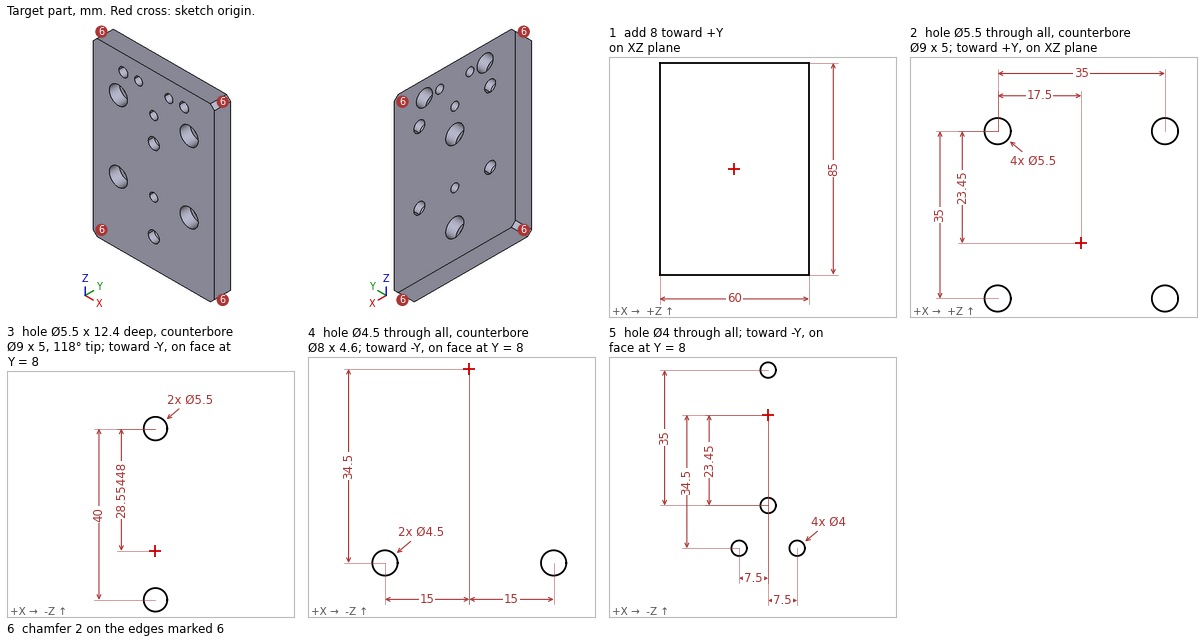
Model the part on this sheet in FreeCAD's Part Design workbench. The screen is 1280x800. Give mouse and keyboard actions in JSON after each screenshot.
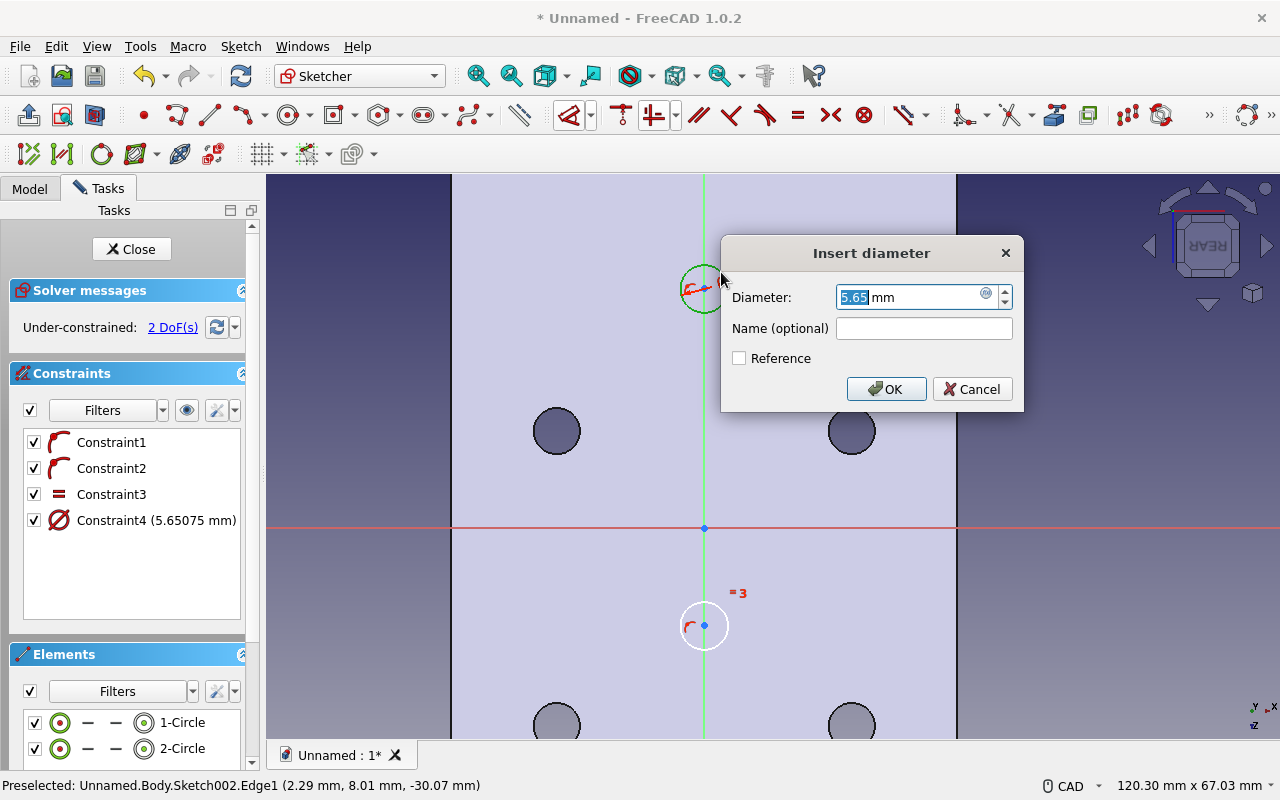
{"action": "type", "text": "5.5"}
{"action": "key", "text": "Return"}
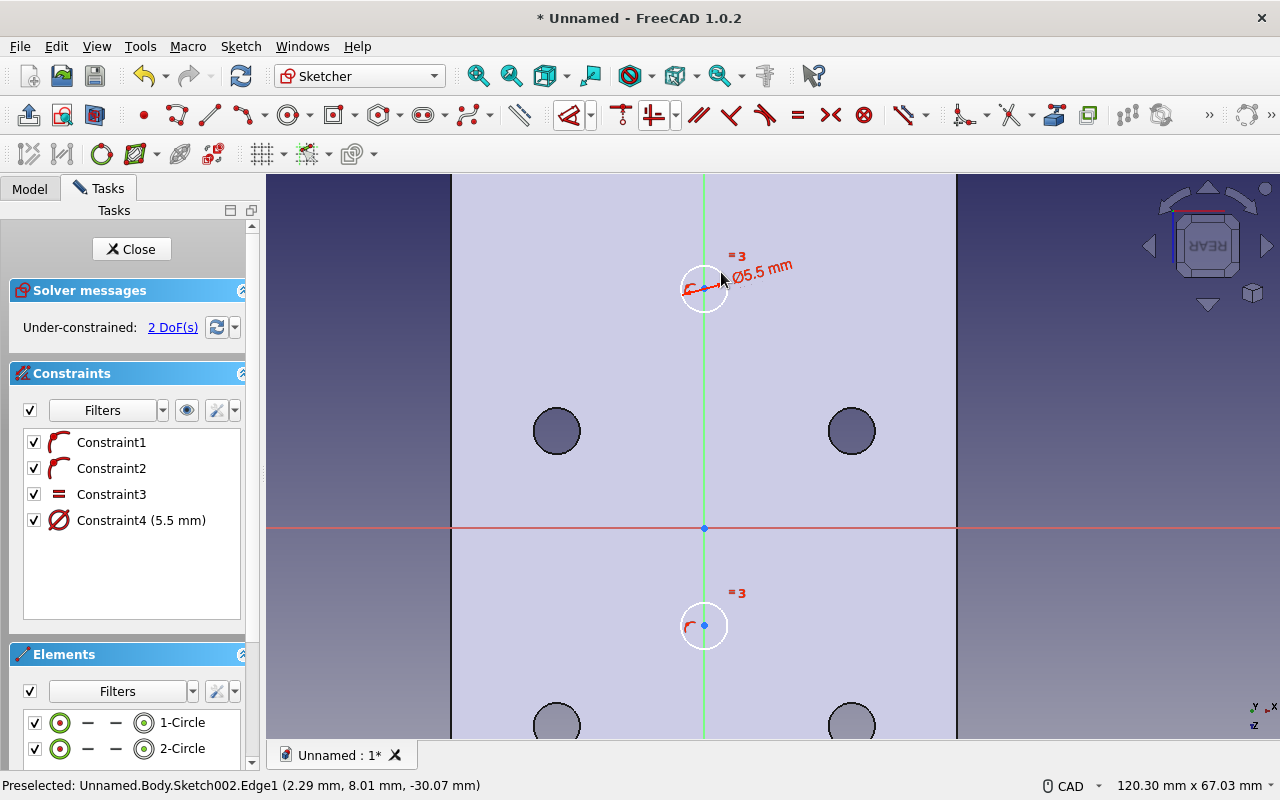
{"action": "left_click", "coordinate": [704, 289]}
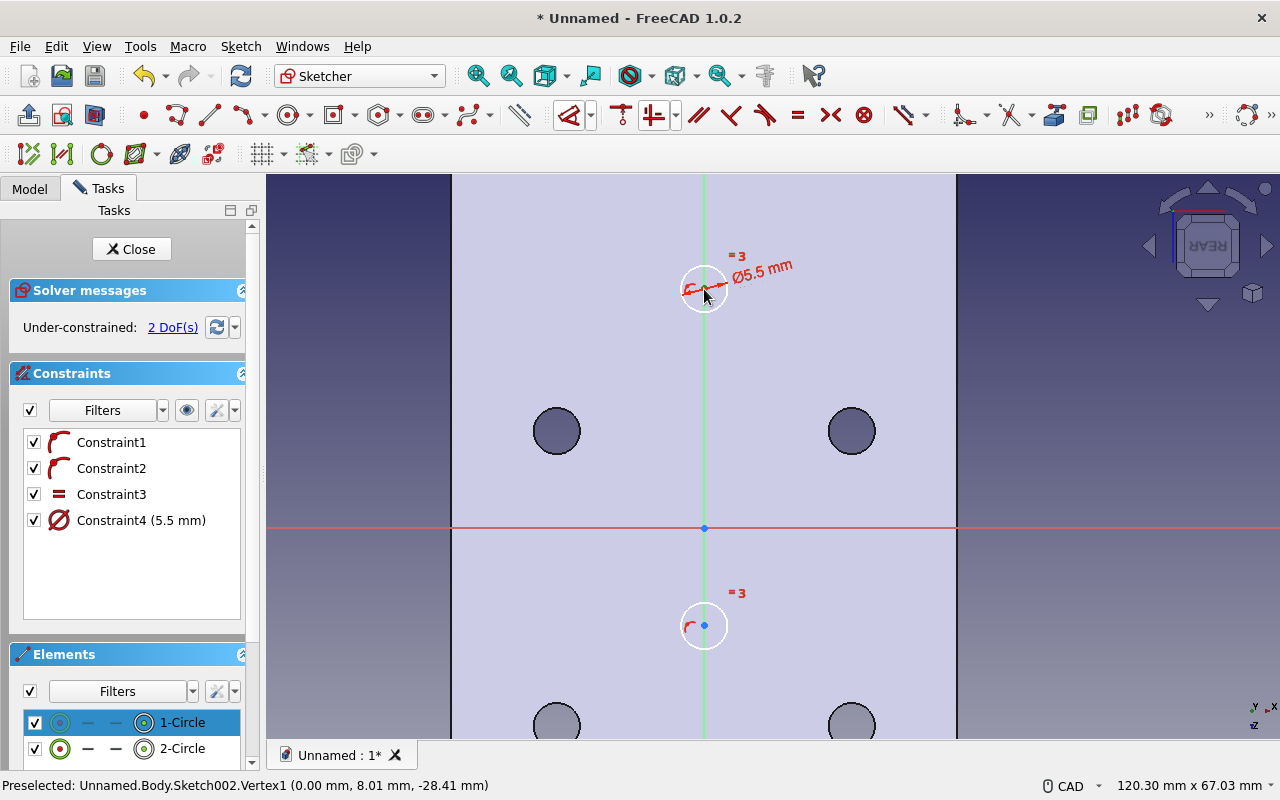
{"action": "left_click", "coordinate": [704, 626]}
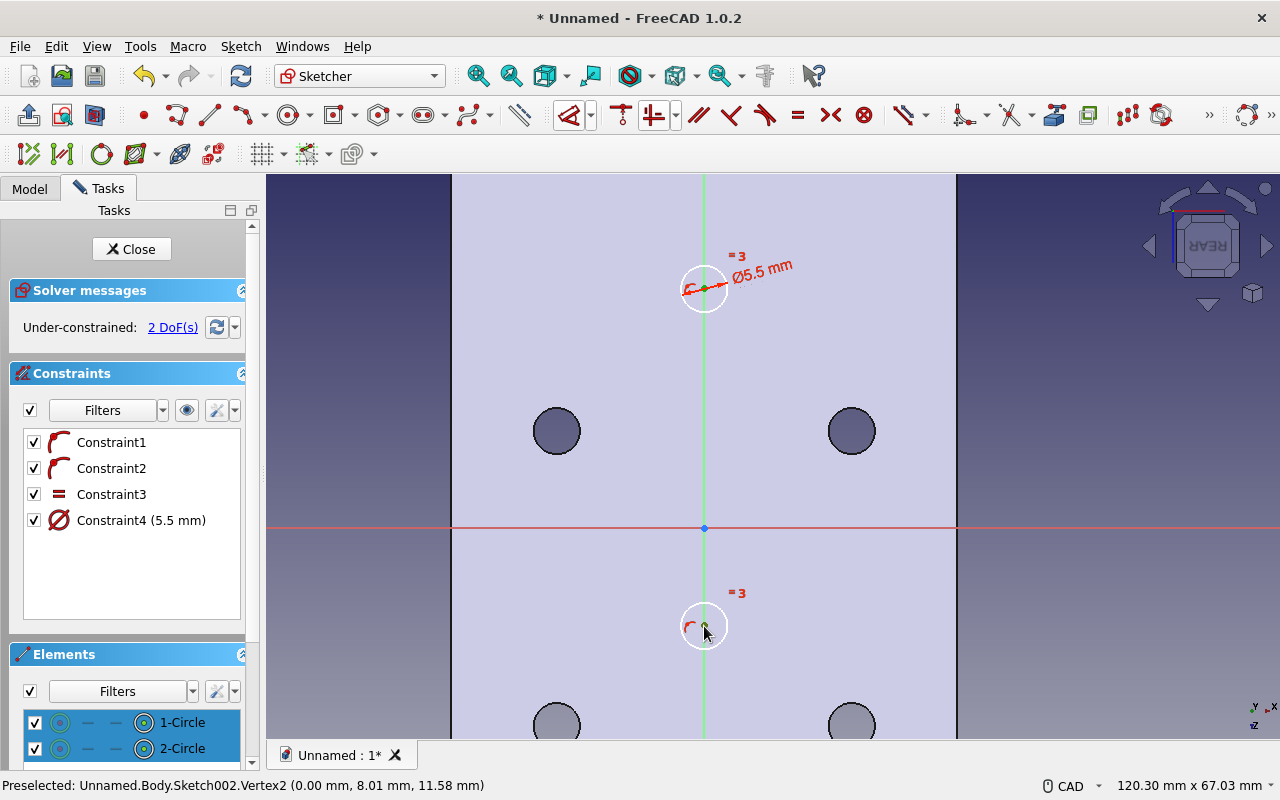
{"action": "left_click", "coordinate": [590, 116]}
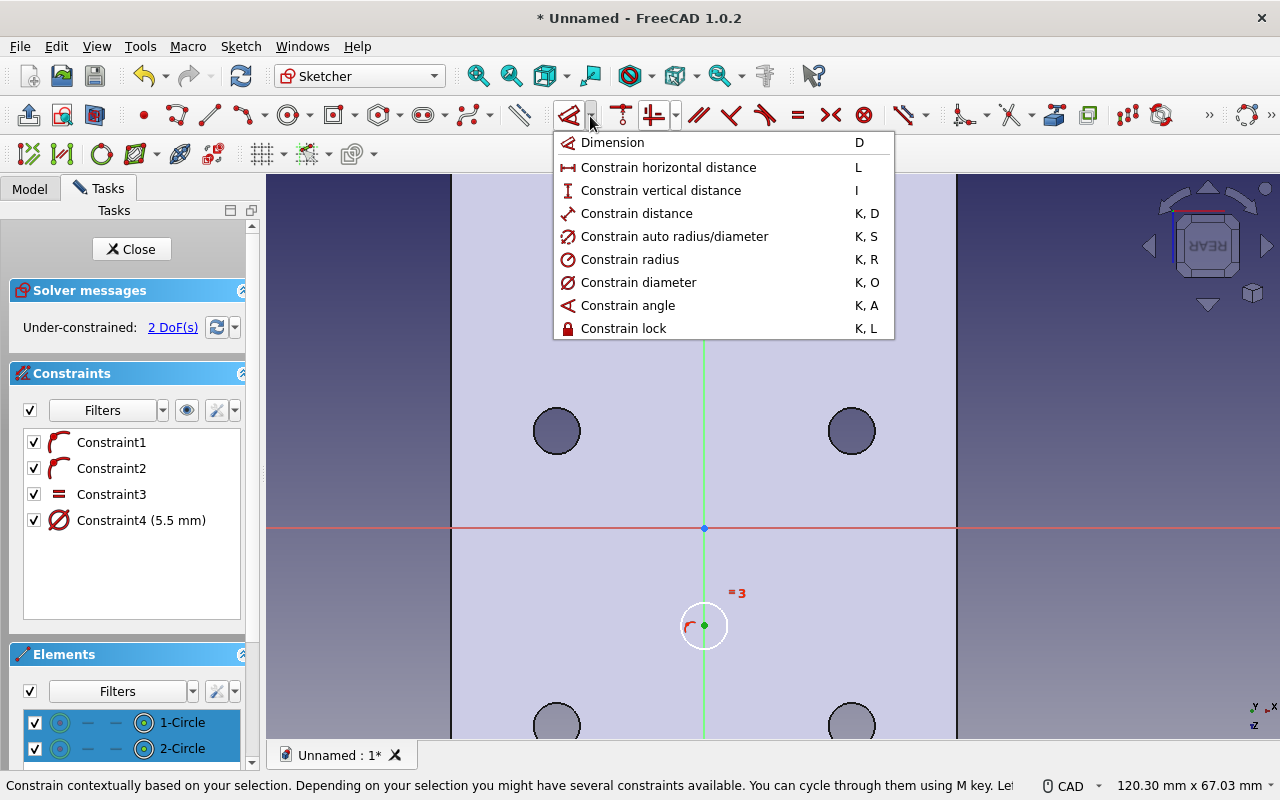
{"action": "left_click", "coordinate": [724, 190]}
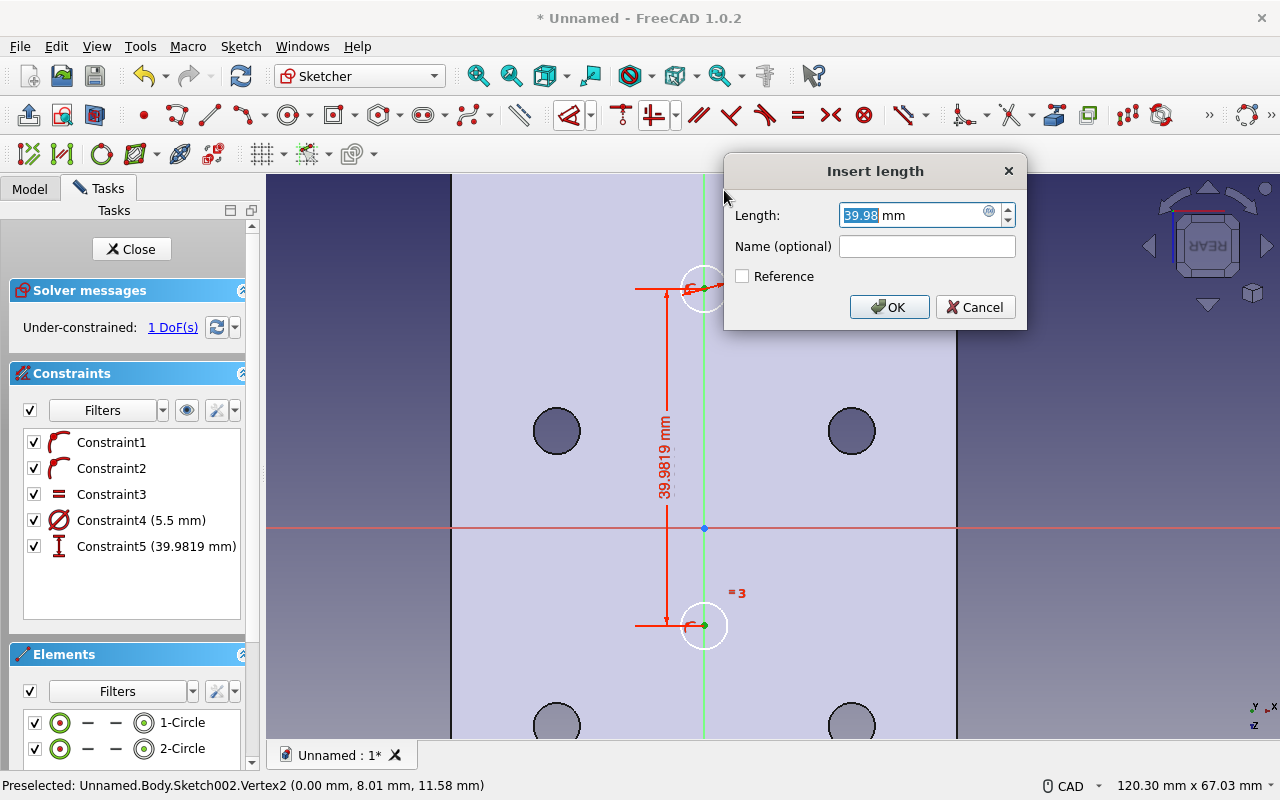
{"action": "type", "text": "40"}
{"action": "key", "text": "Return"}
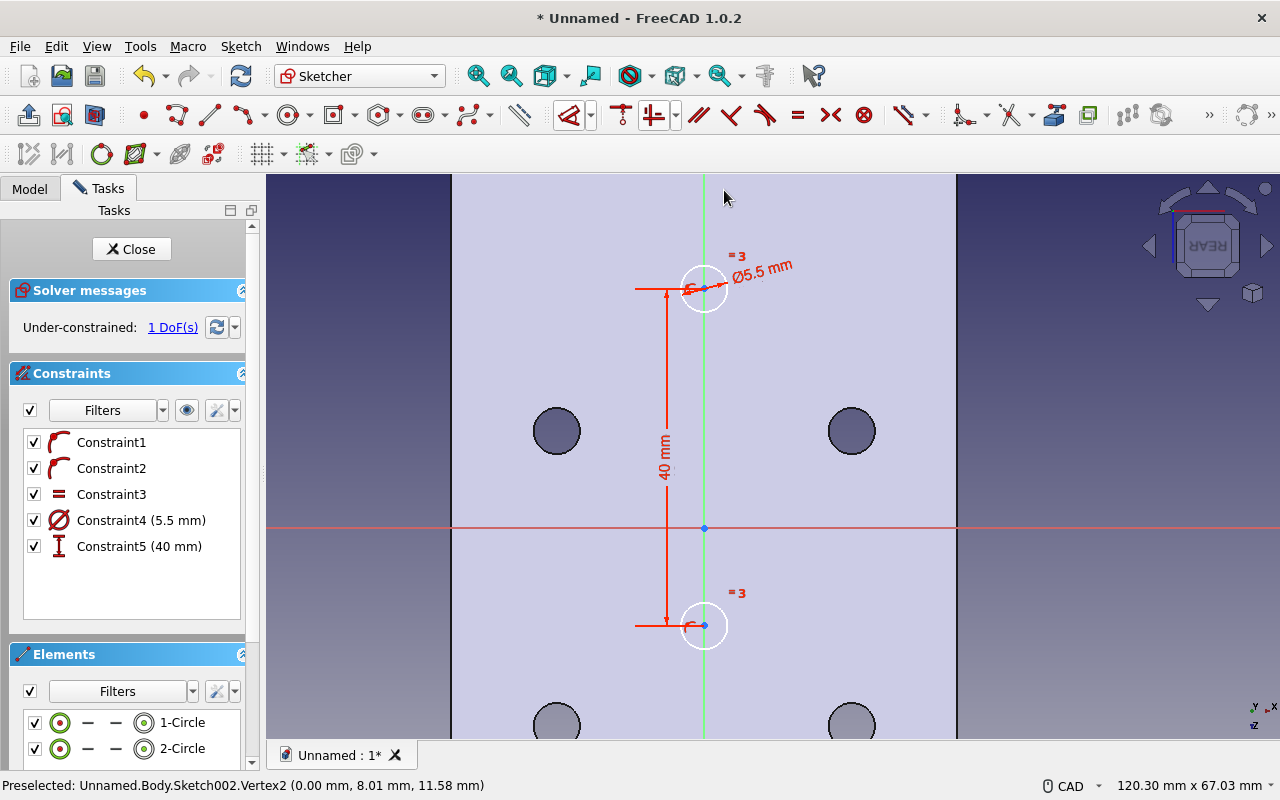
{"action": "left_click", "coordinate": [704, 289]}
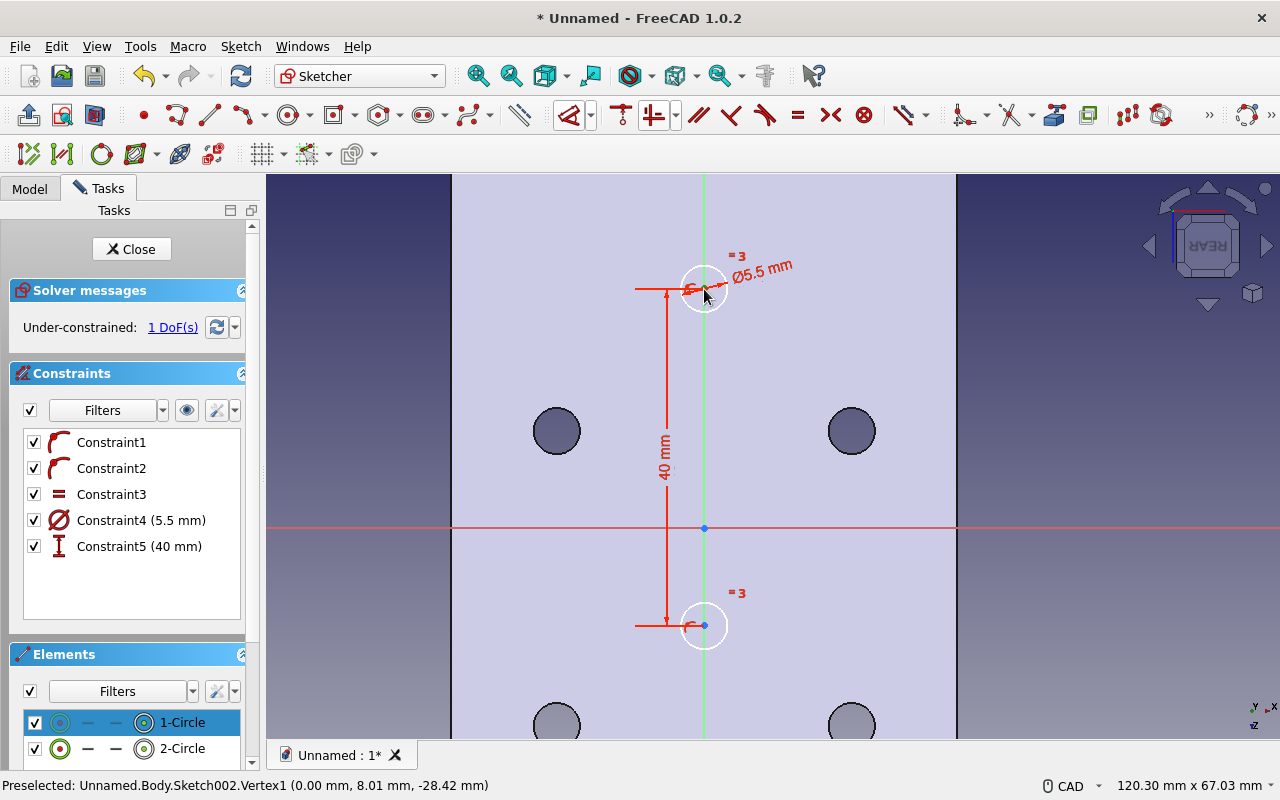
{"action": "key", "text": "i"}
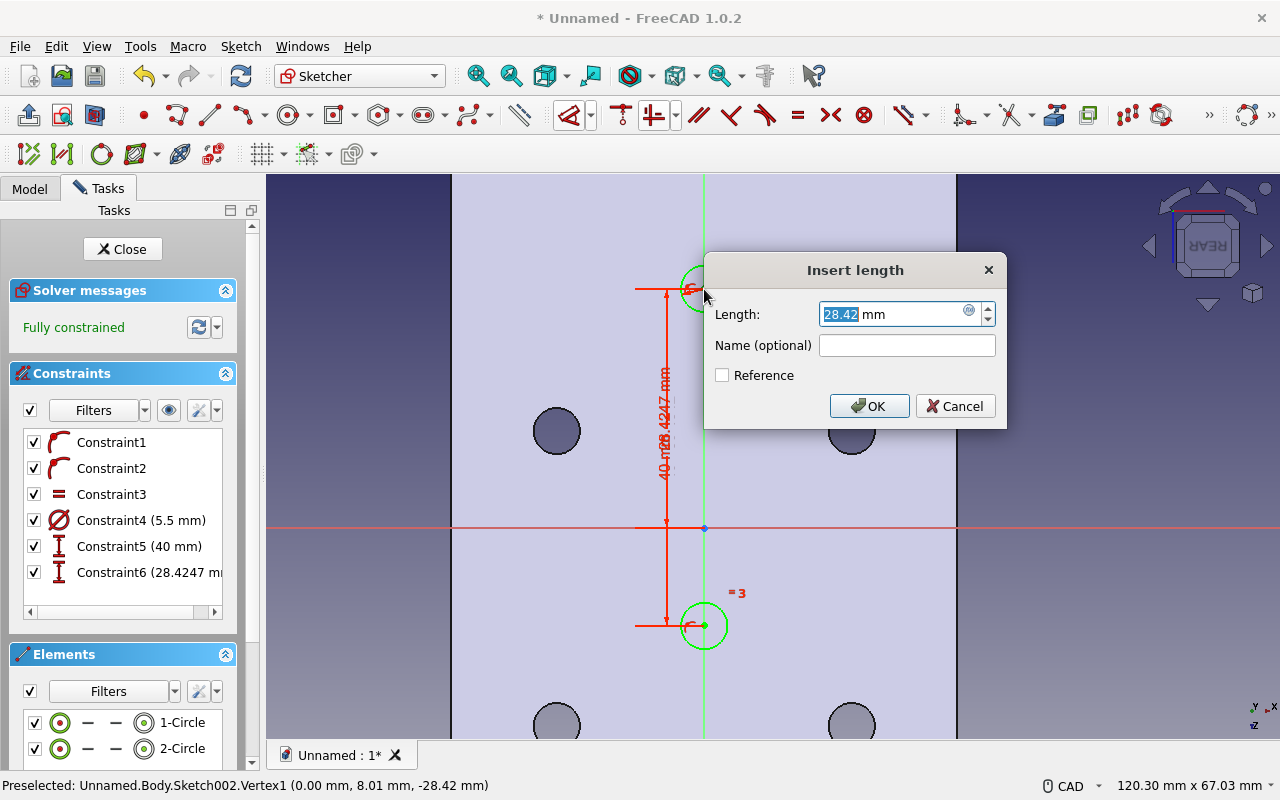
{"action": "type", "text": "28.55448"}
{"action": "key", "text": "Return"}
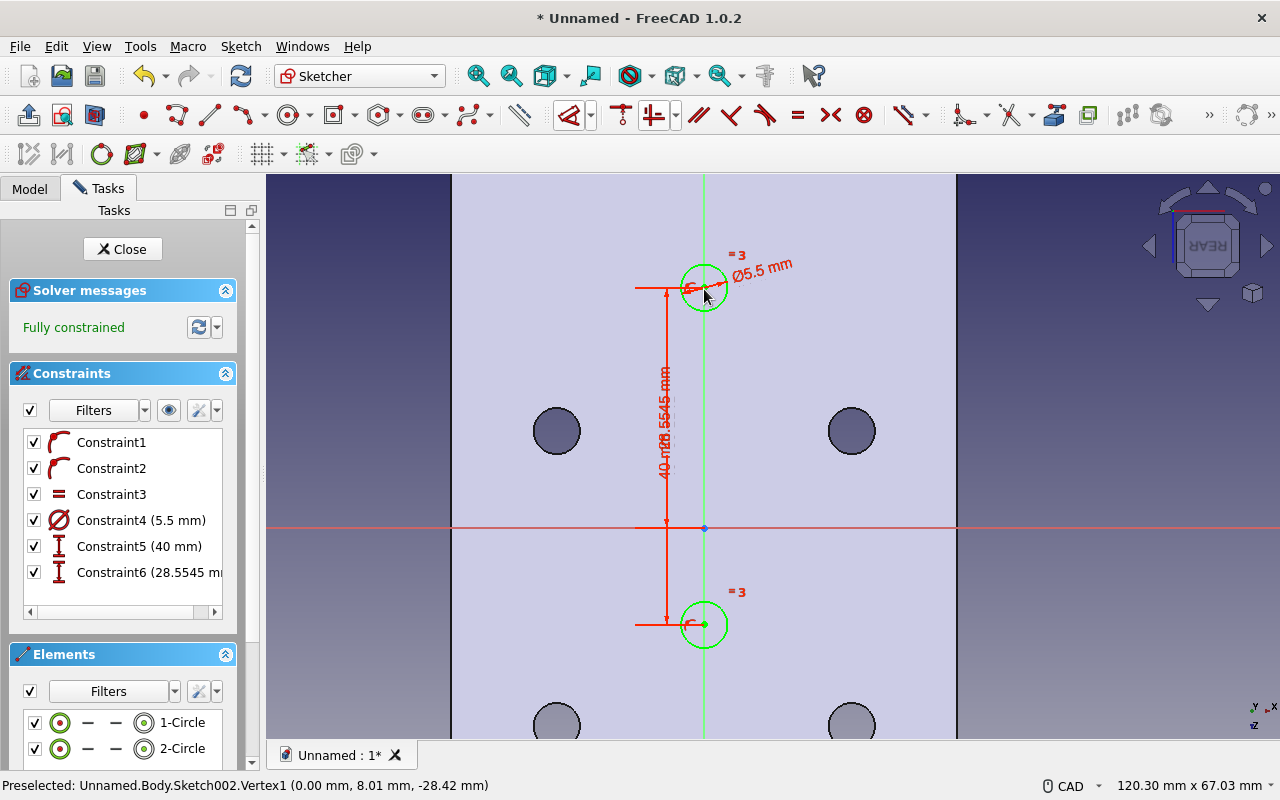
{"action": "left_click", "coordinate": [123, 249]}